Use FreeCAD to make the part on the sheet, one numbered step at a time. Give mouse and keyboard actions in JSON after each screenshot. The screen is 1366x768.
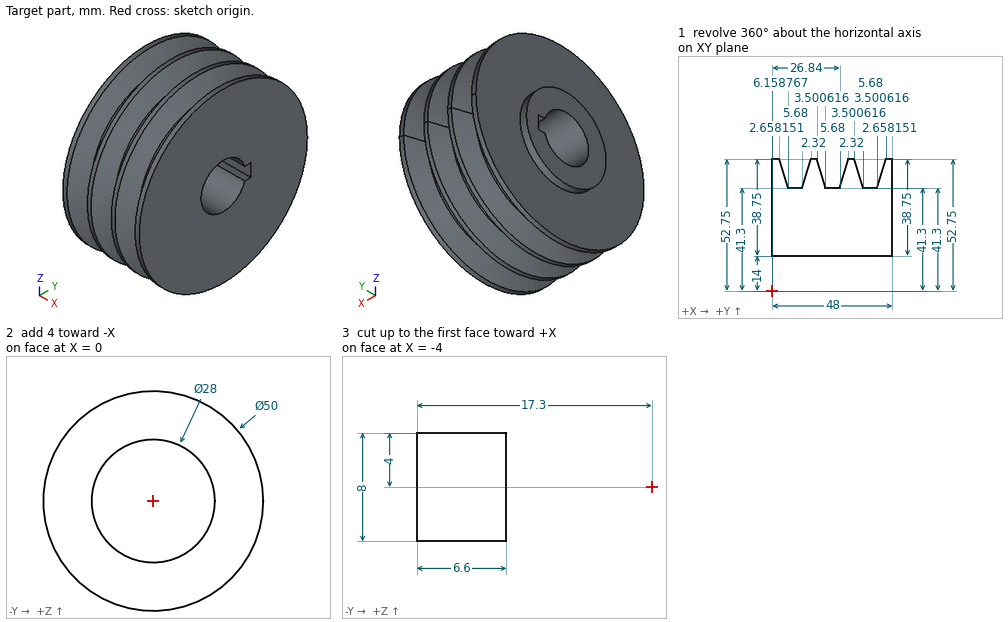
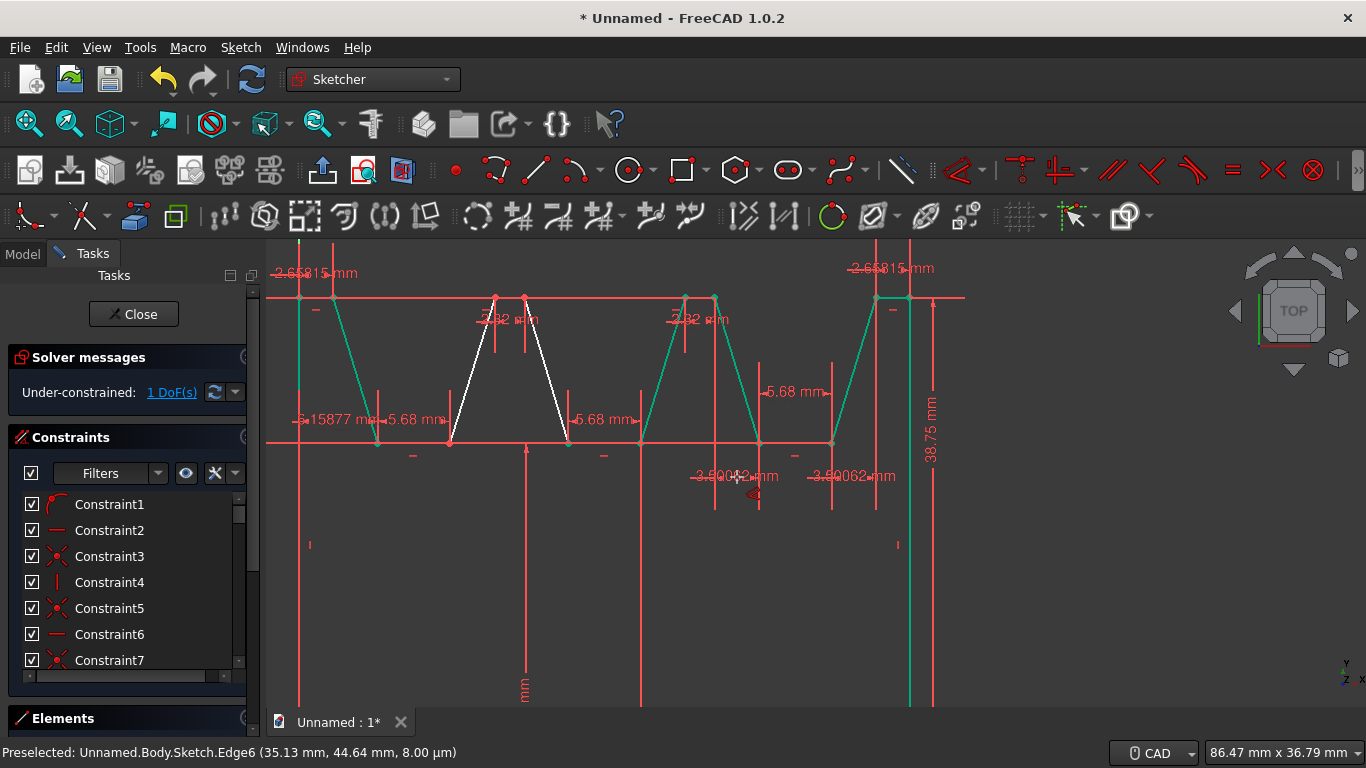
{"action": "left_click", "coordinate": [555, 400]}
{"action": "left_click", "coordinate": [547, 477]}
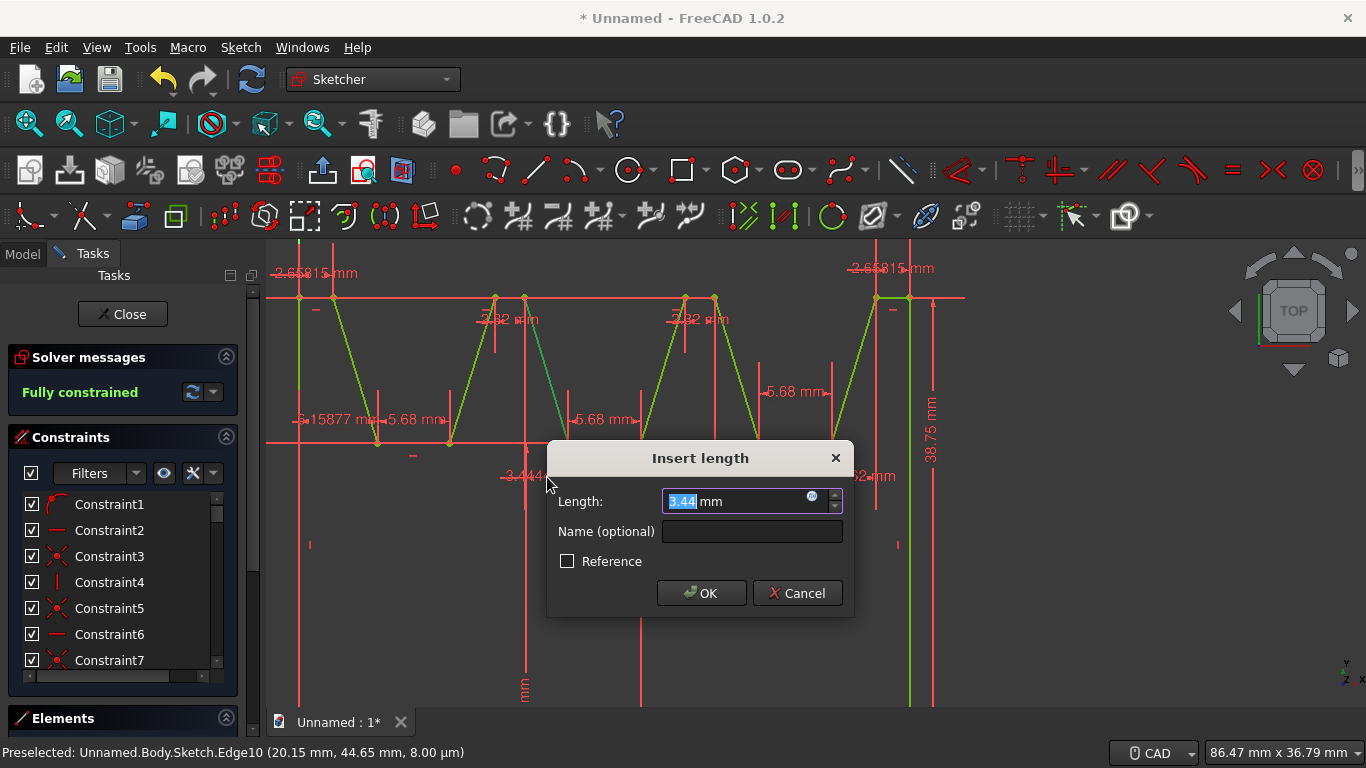
{"action": "type", "text": "3.500616"}
{"action": "key", "text": "Return"}
{"action": "key", "text": "Escape"}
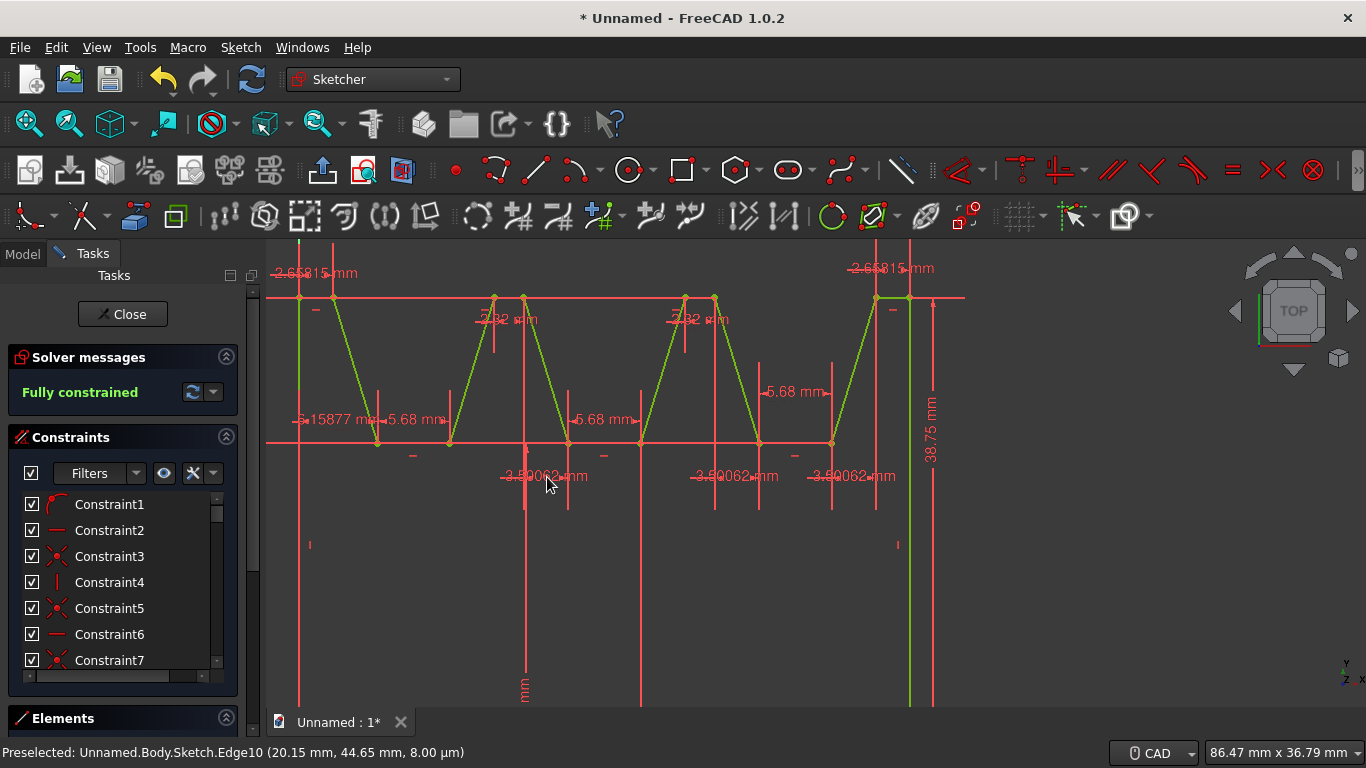
{"action": "left_click", "coordinate": [123, 314]}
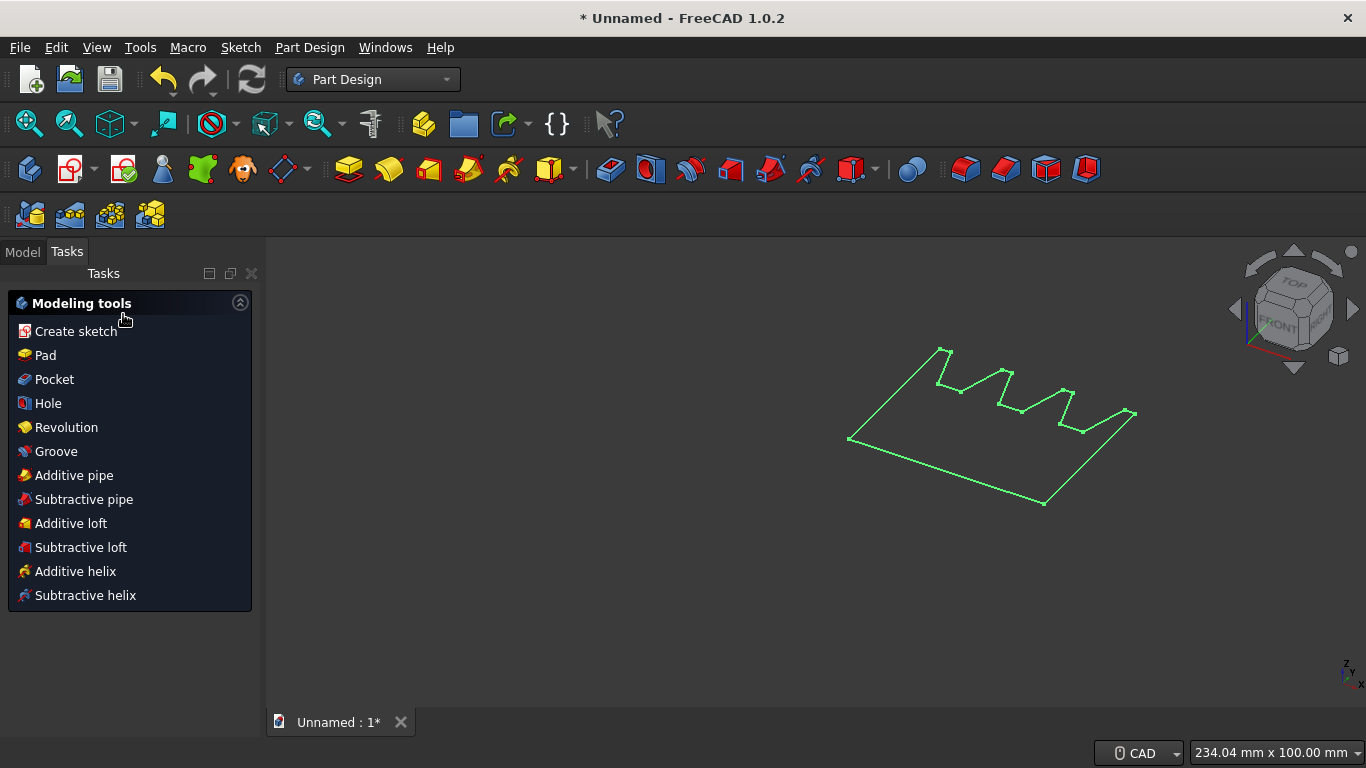
{"action": "left_click", "coordinate": [390, 170]}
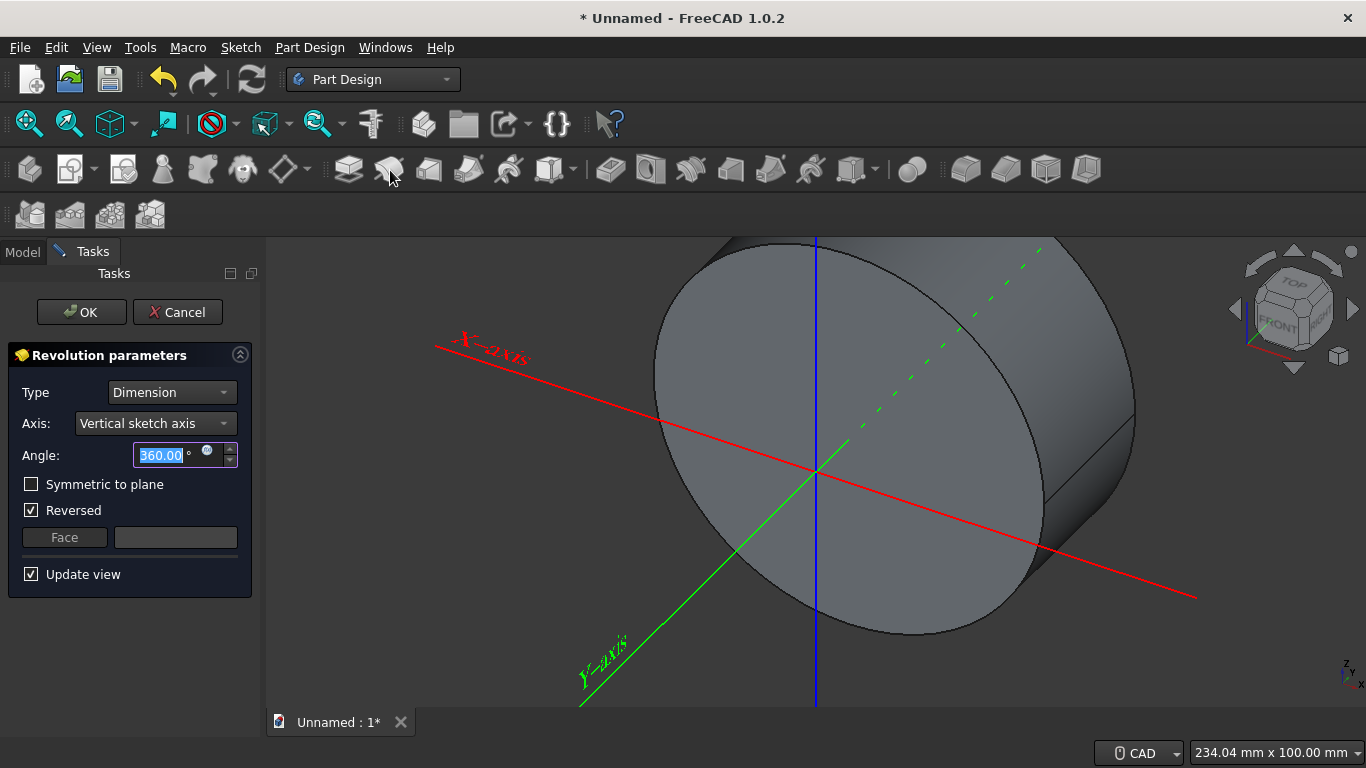
{"action": "left_click", "coordinate": [156, 424]}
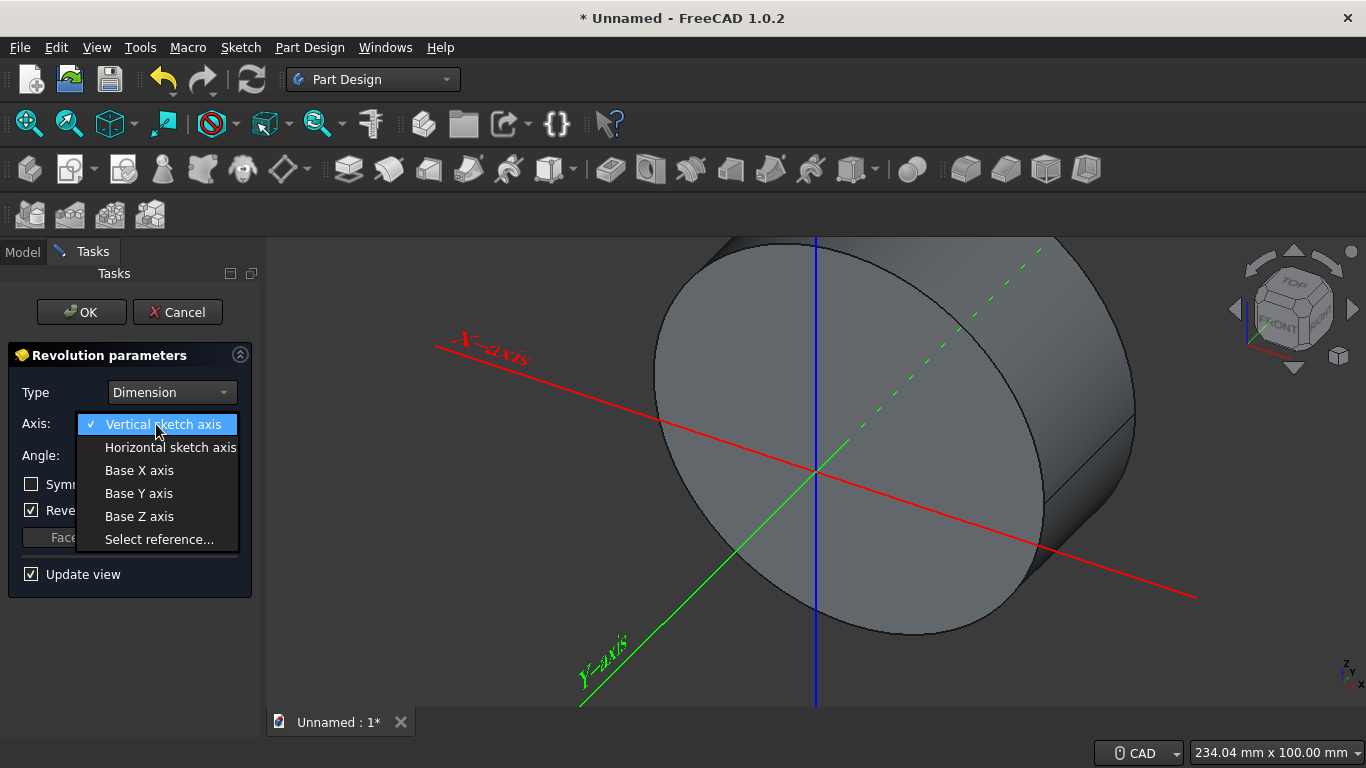
{"action": "left_click", "coordinate": [156, 448]}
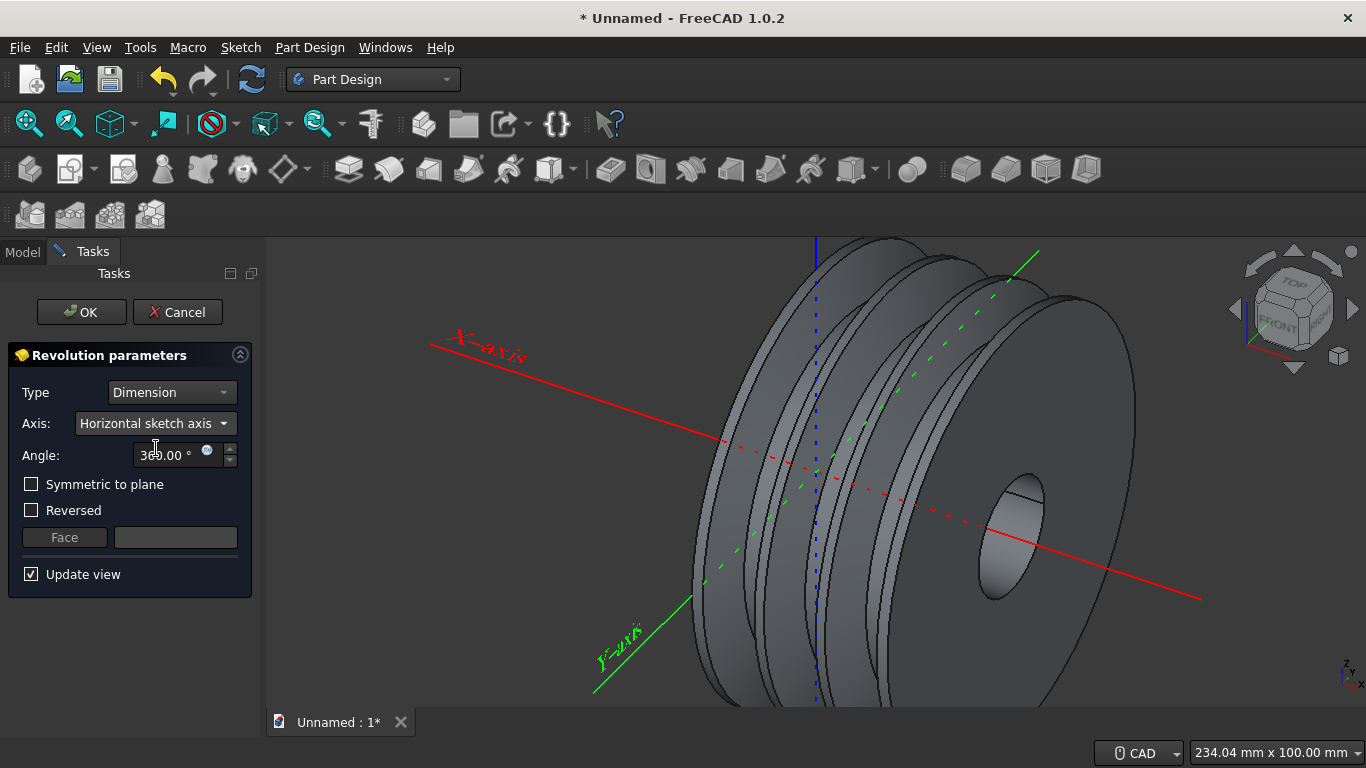
{"action": "left_click", "coordinate": [82, 312]}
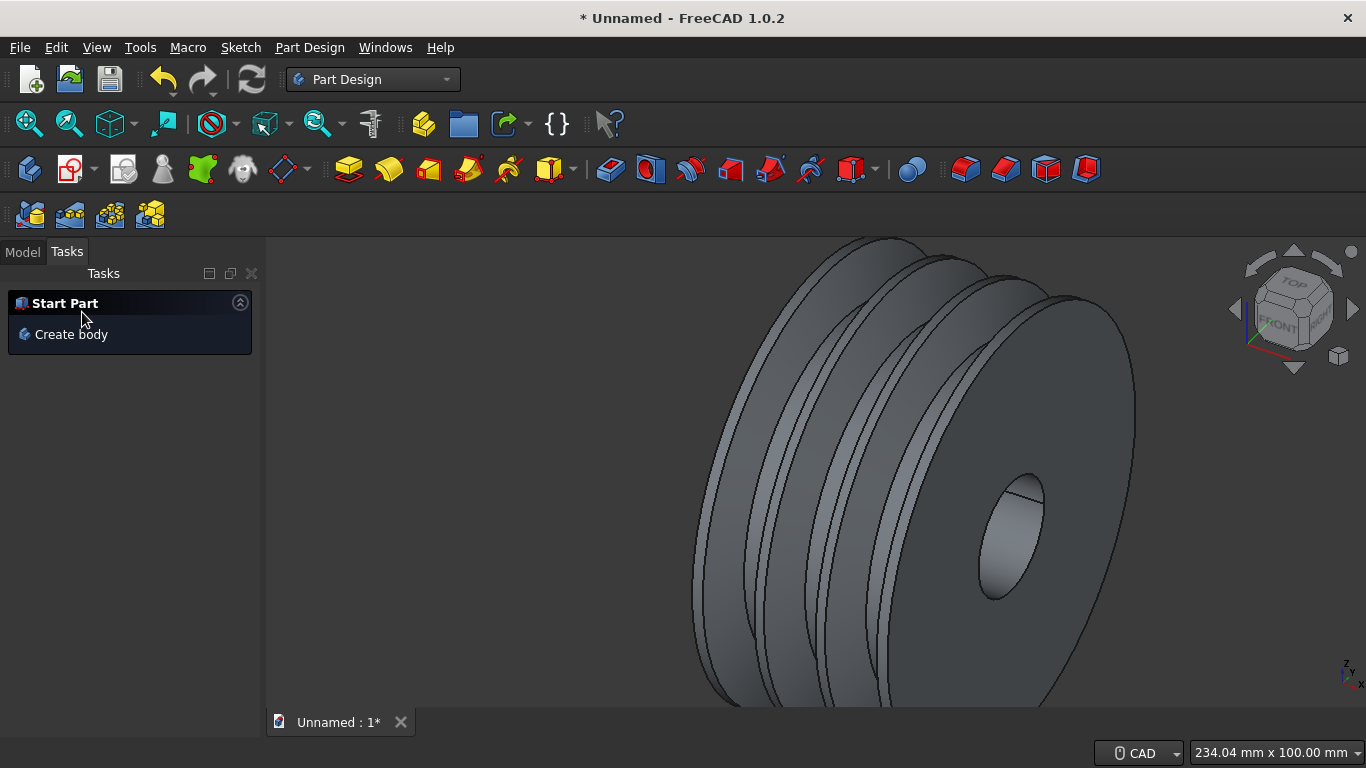
{"action": "left_click", "coordinate": [30, 124]}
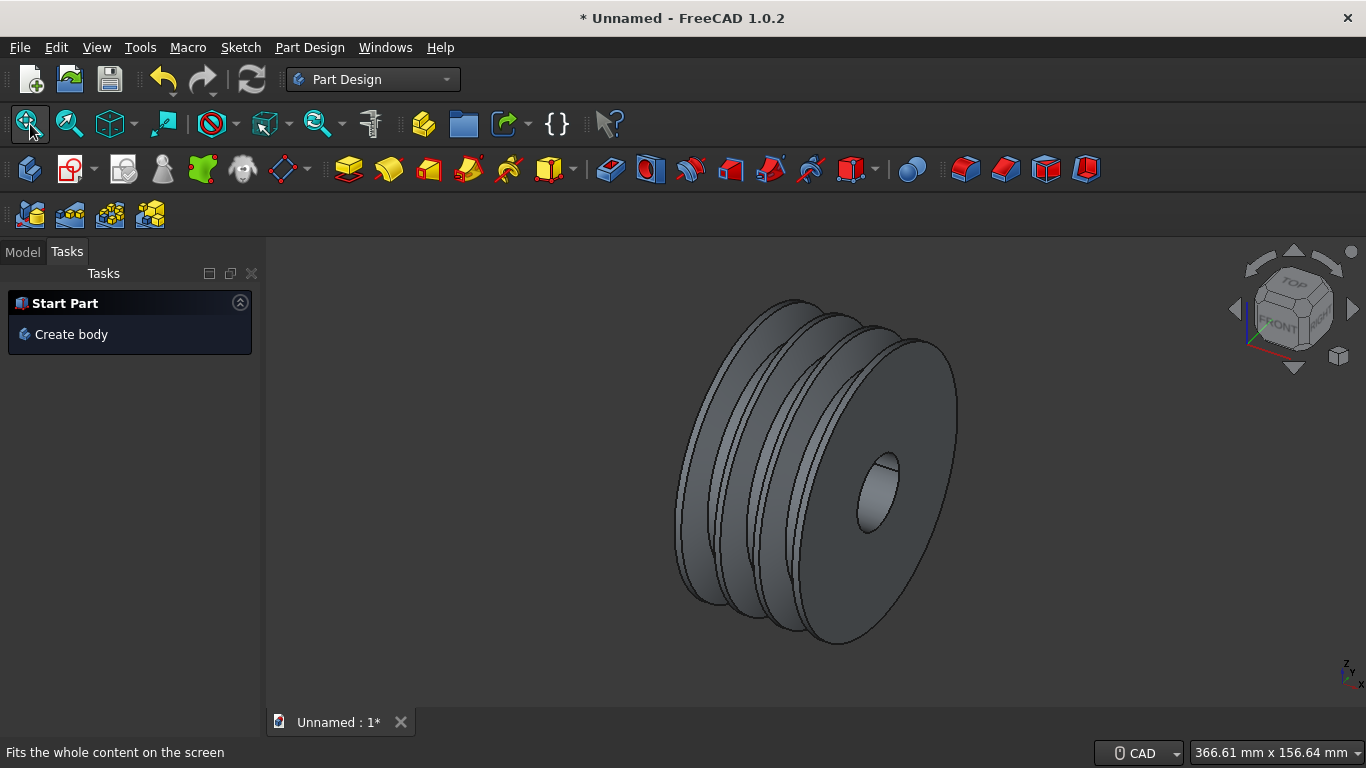
{"action": "key", "text": "6"}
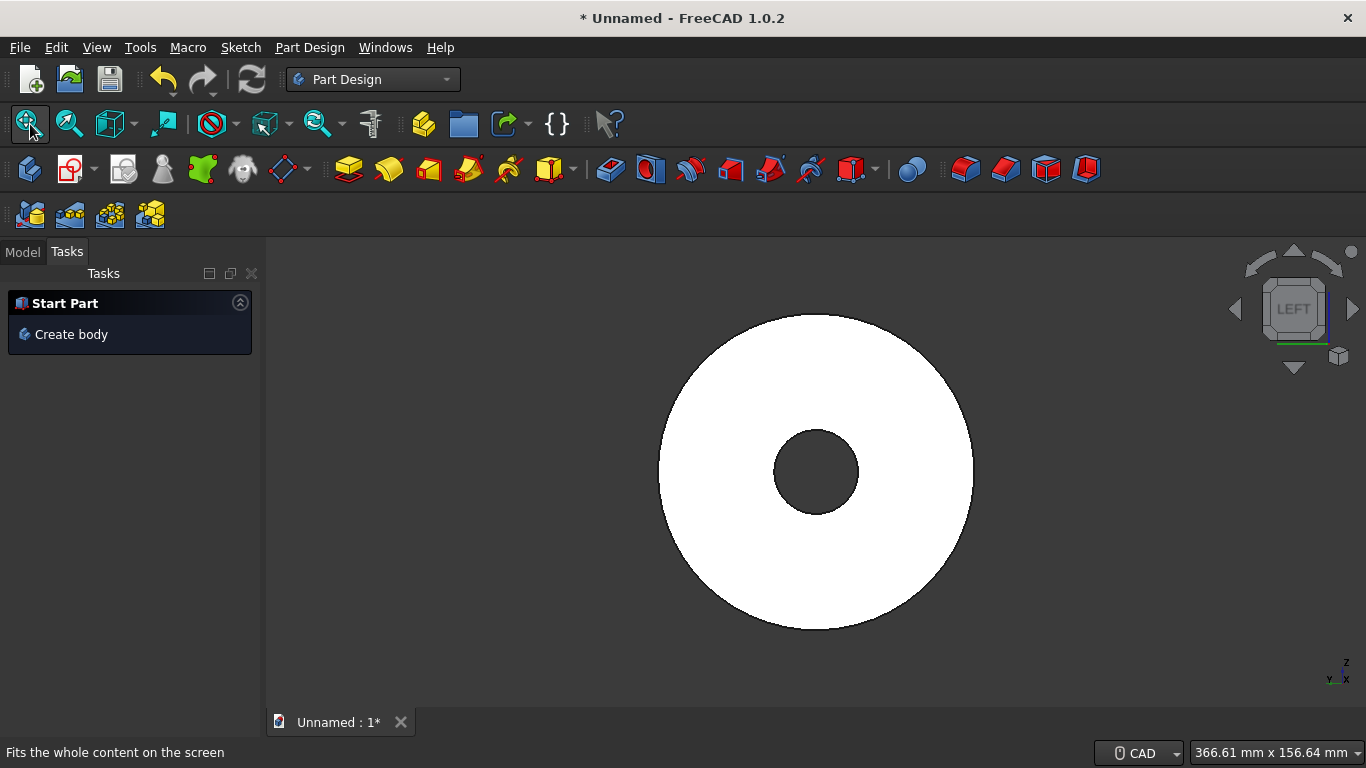
{"action": "left_click", "coordinate": [726, 426]}